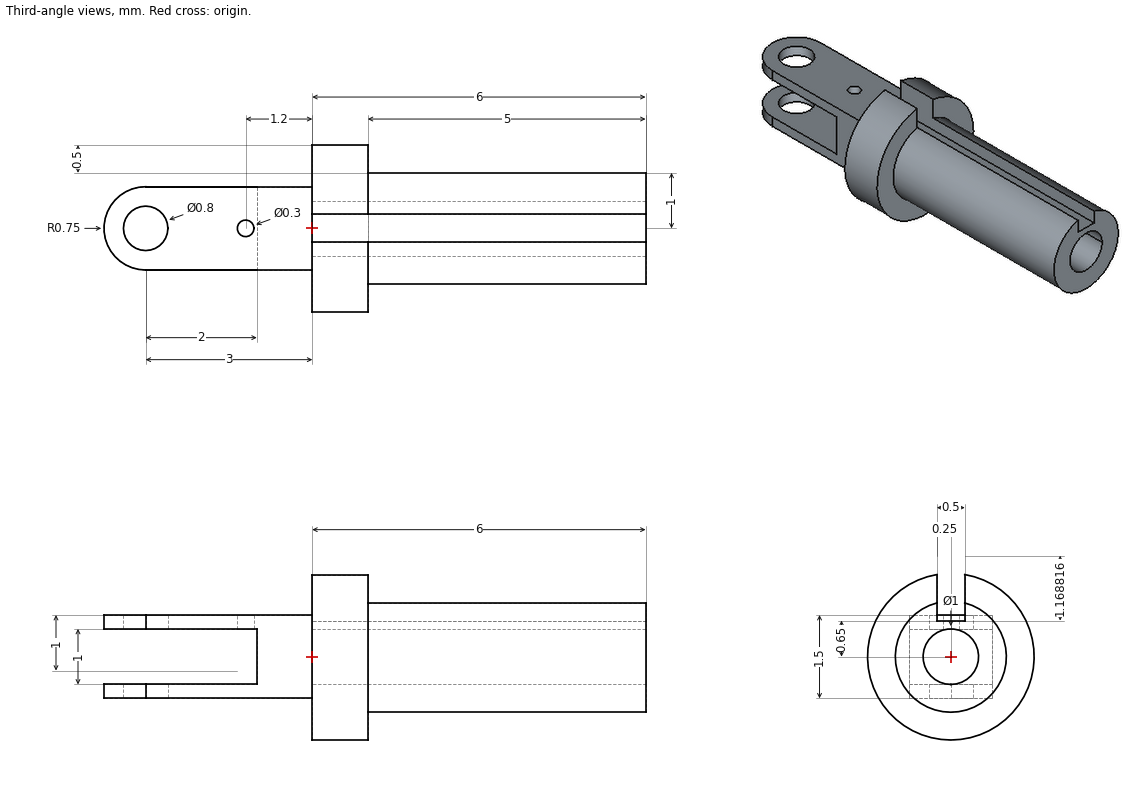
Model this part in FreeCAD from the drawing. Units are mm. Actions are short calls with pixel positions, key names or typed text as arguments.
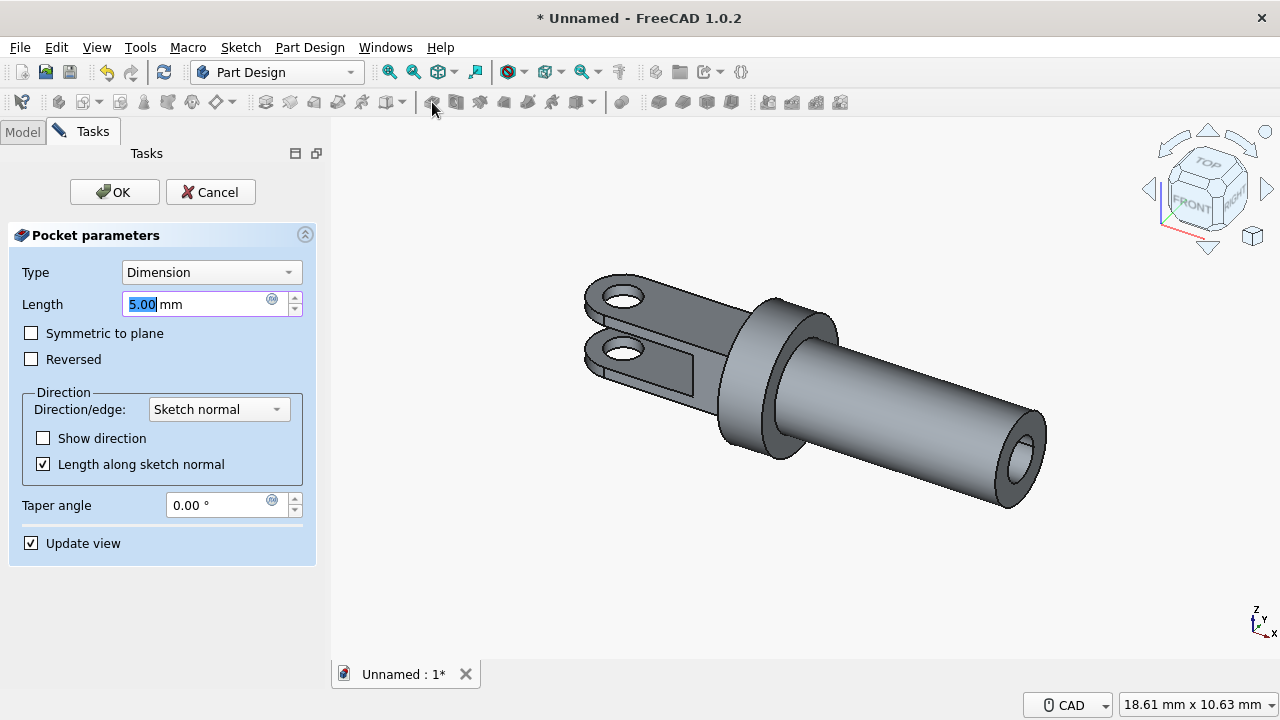
text(6)
key(Tab)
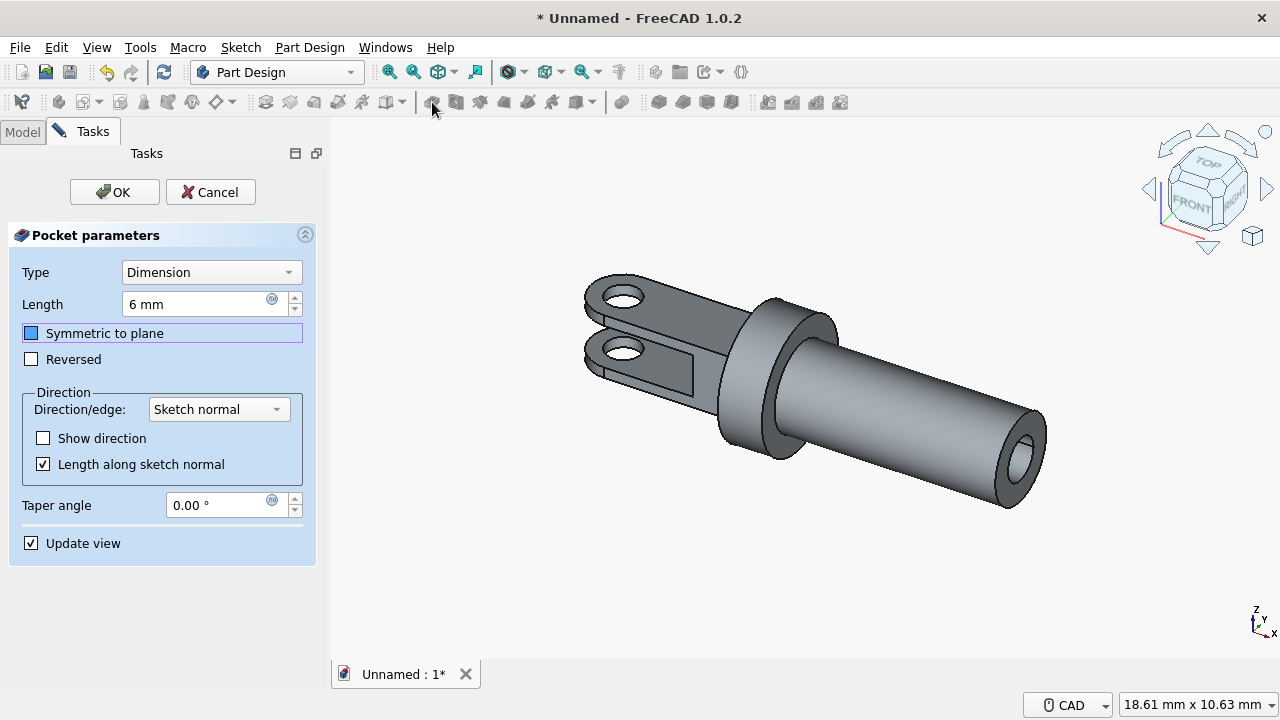
click(115, 192)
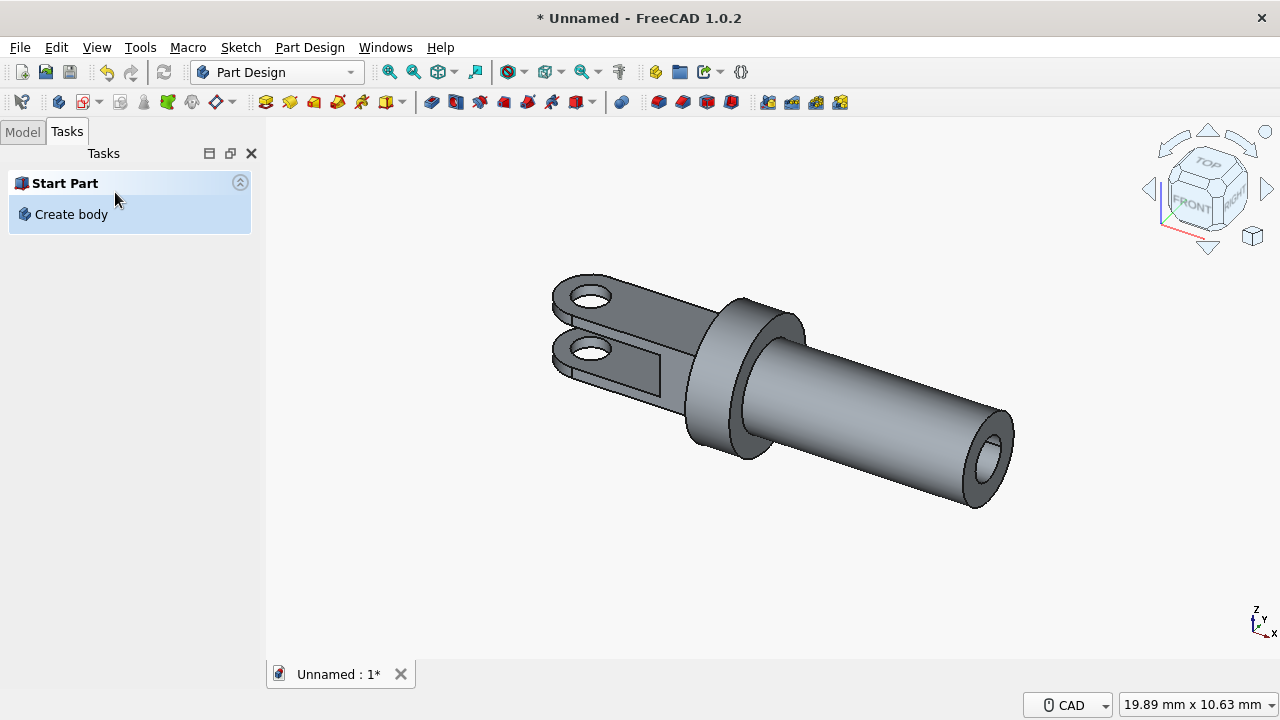
click(1003, 420)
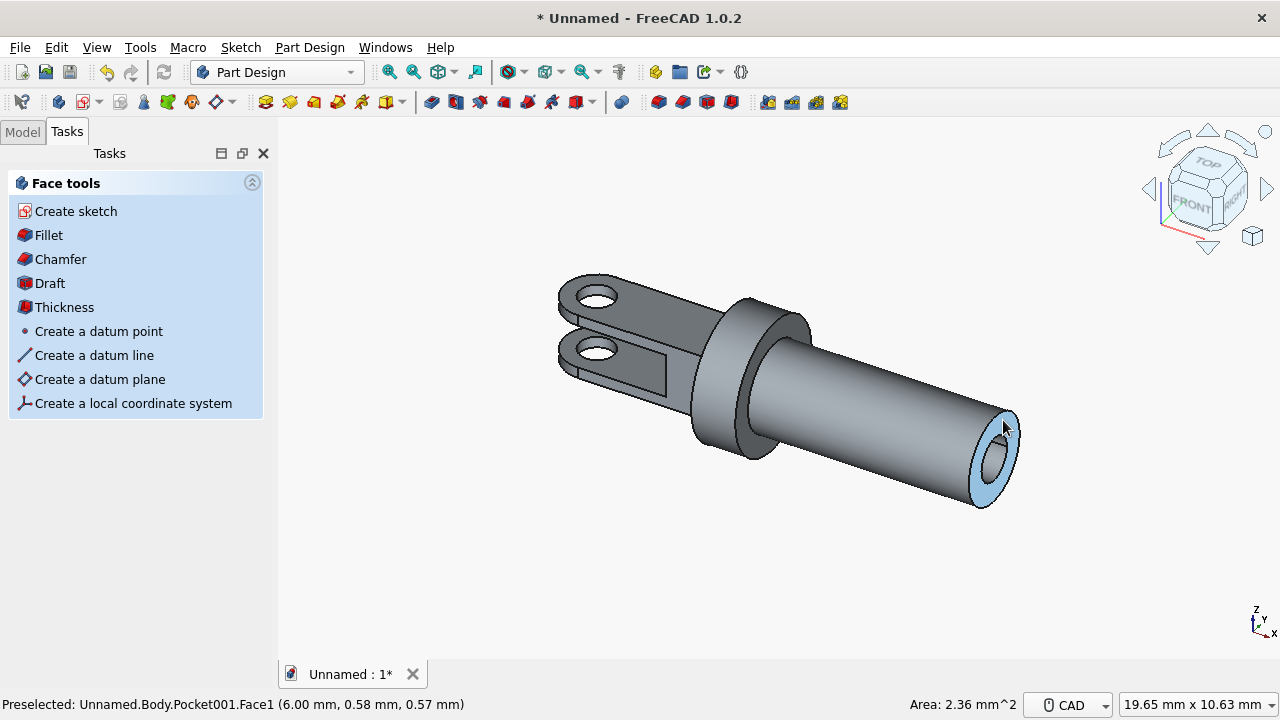
click(84, 102)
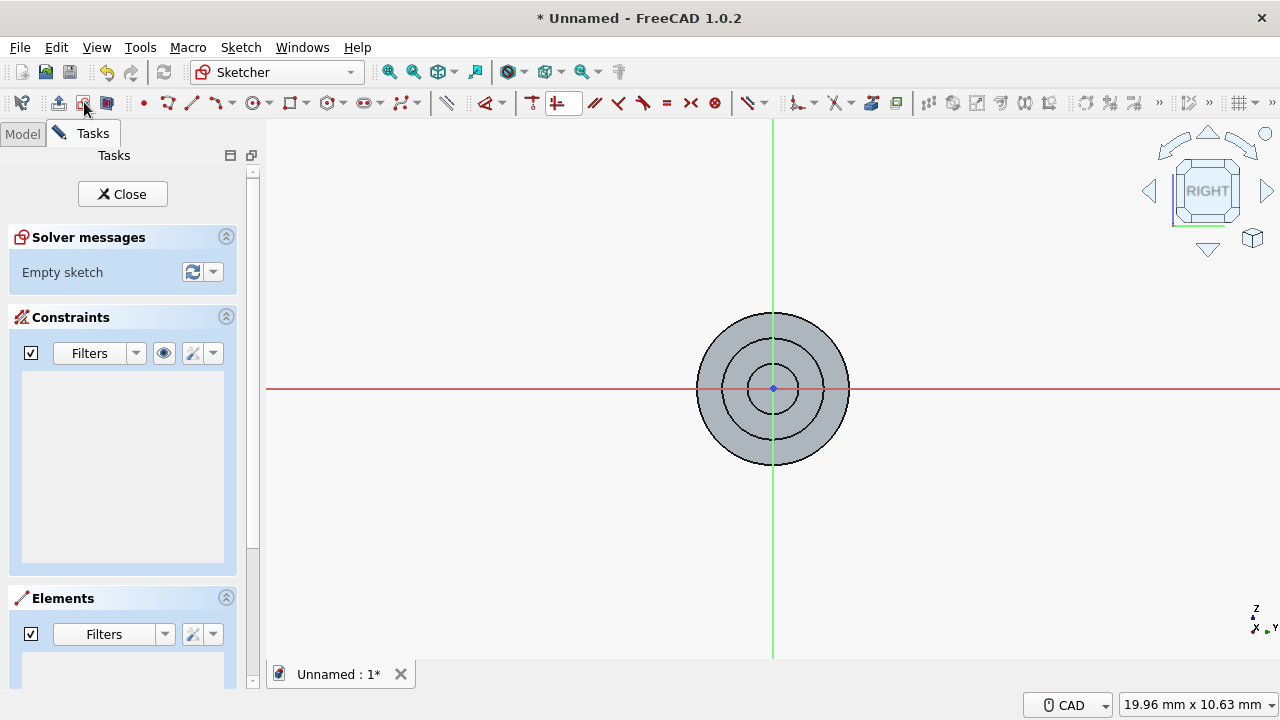
scroll(795, 328, up, 7)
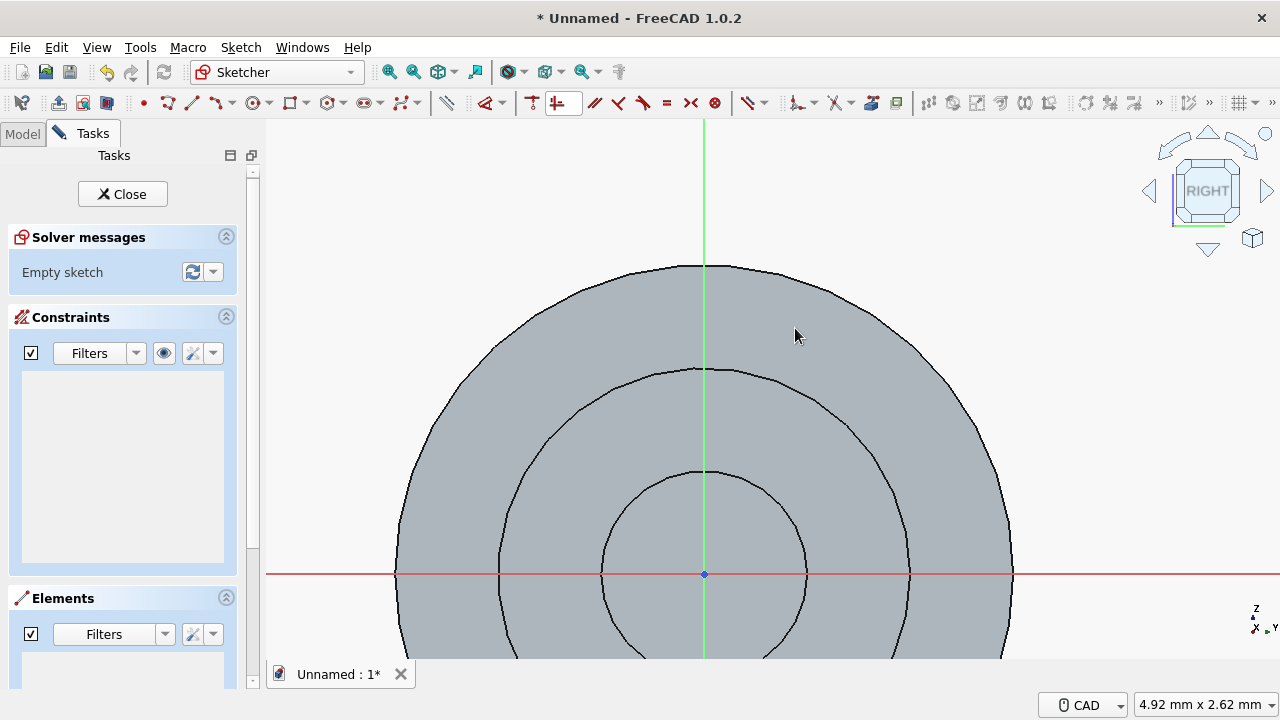
click(290, 104)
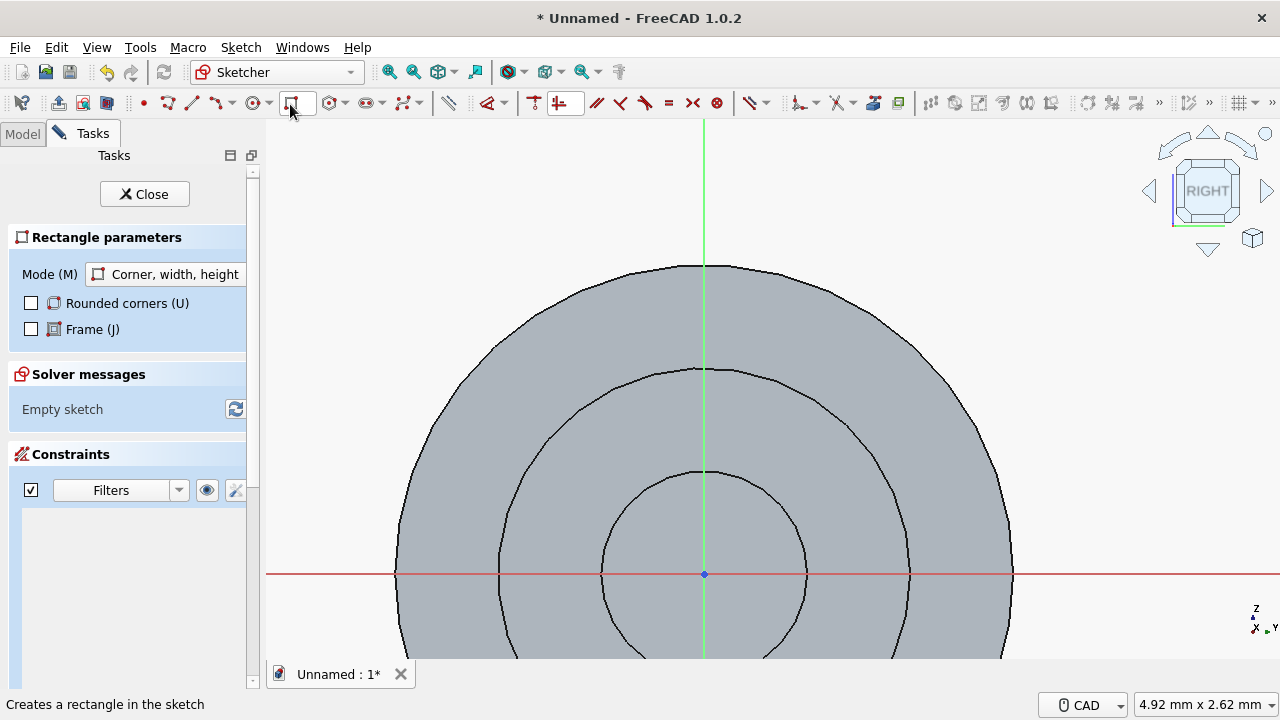
click(653, 200)
move(756, 440)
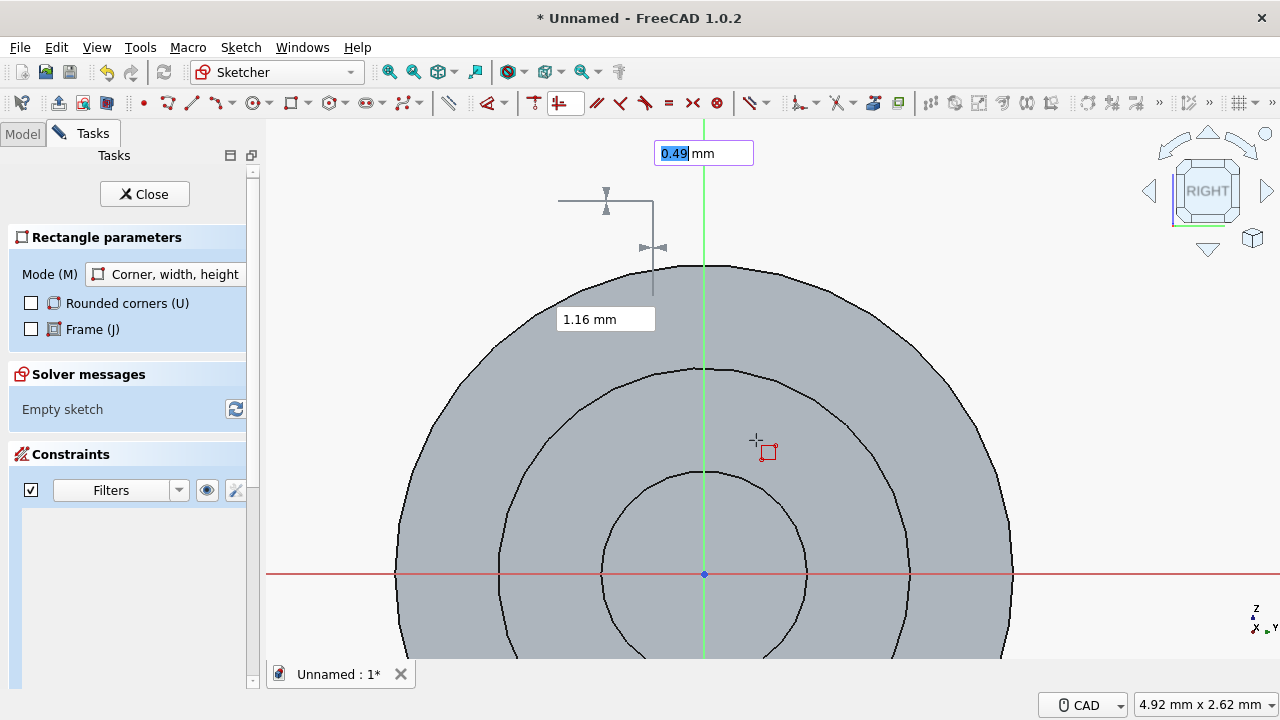
text(0.5)
key(Tab)
text(1.168816)
key(Return)
key(Escape)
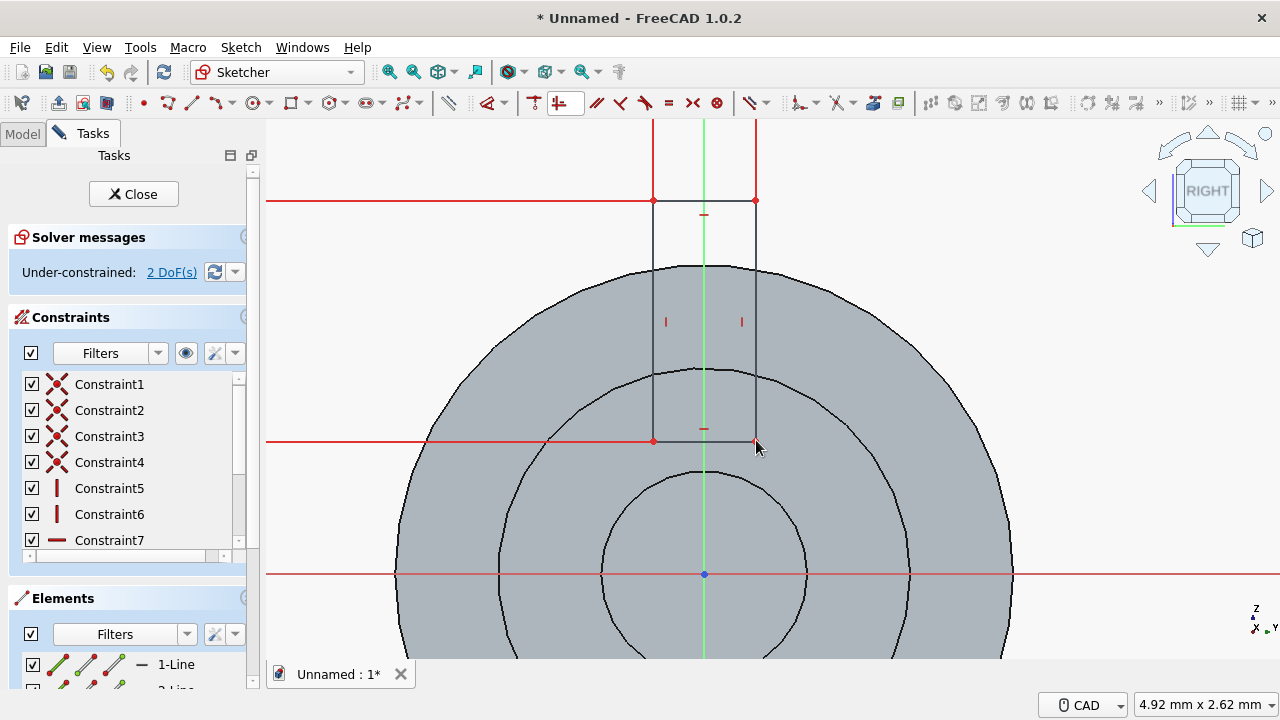
click(488, 104)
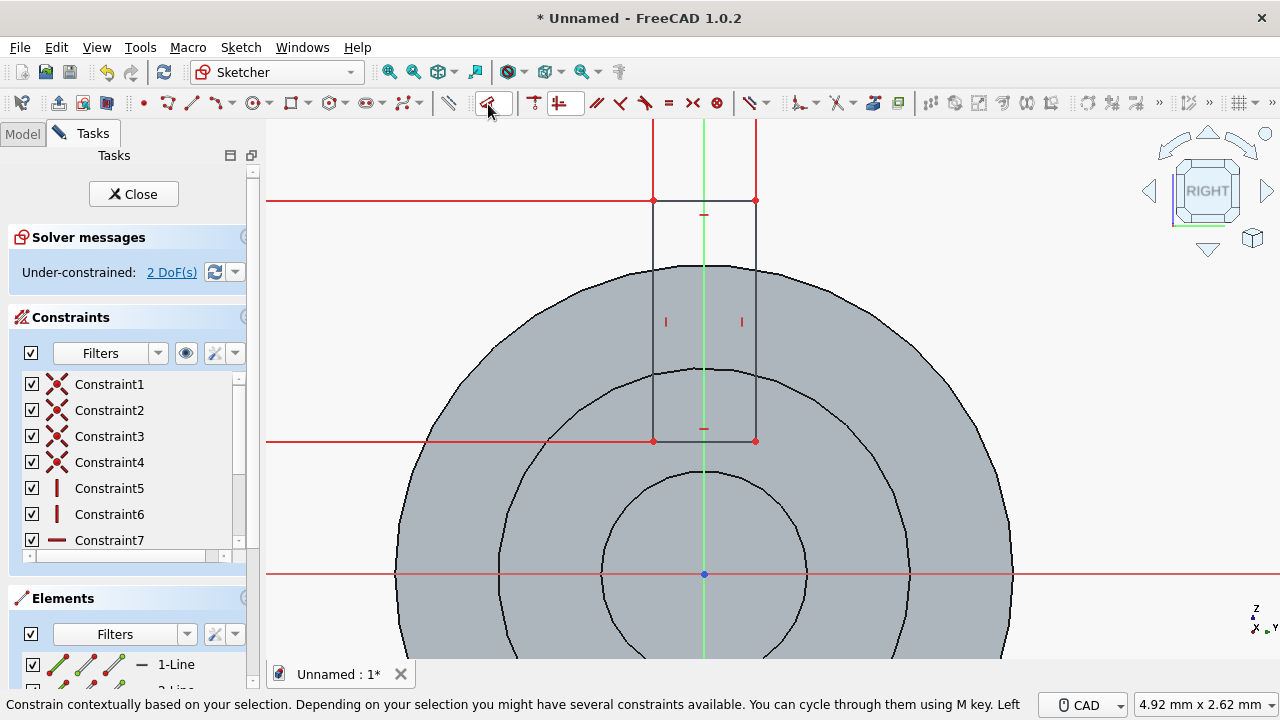
click(653, 201)
click(679, 608)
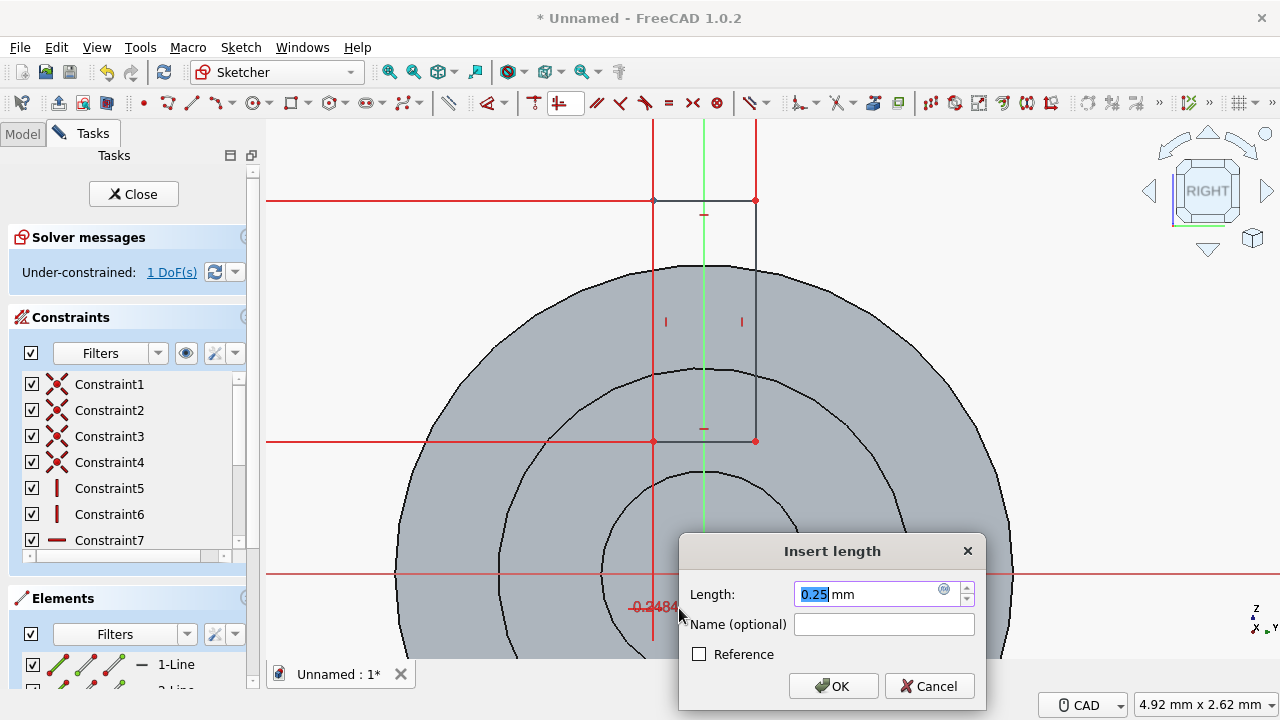
text(0.25)
key(Return)